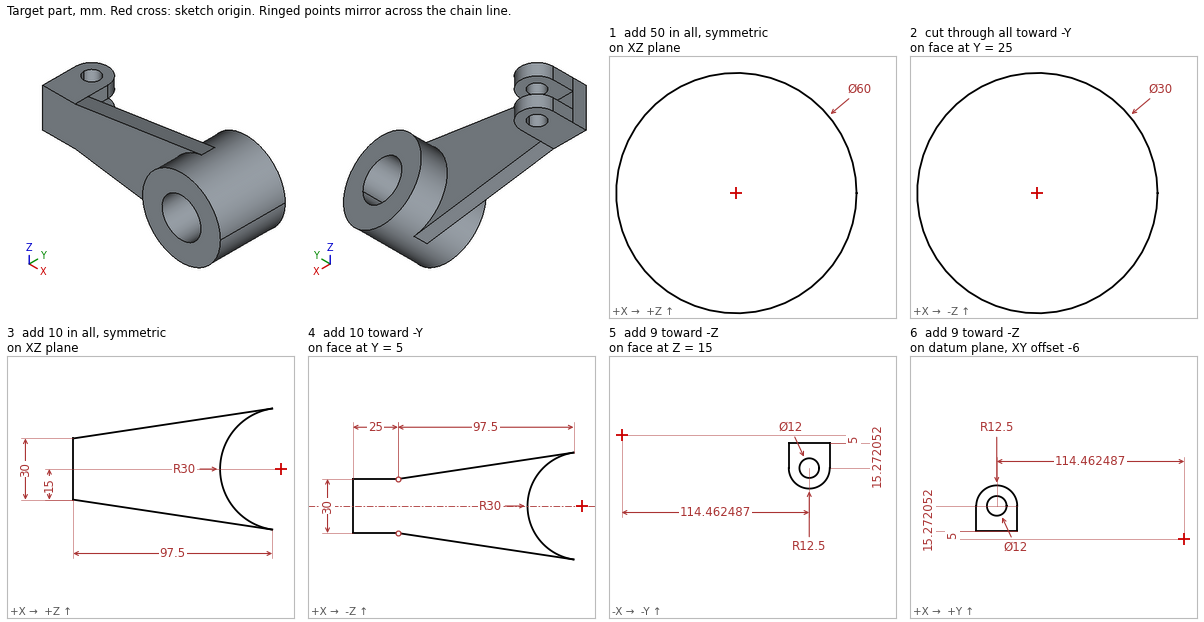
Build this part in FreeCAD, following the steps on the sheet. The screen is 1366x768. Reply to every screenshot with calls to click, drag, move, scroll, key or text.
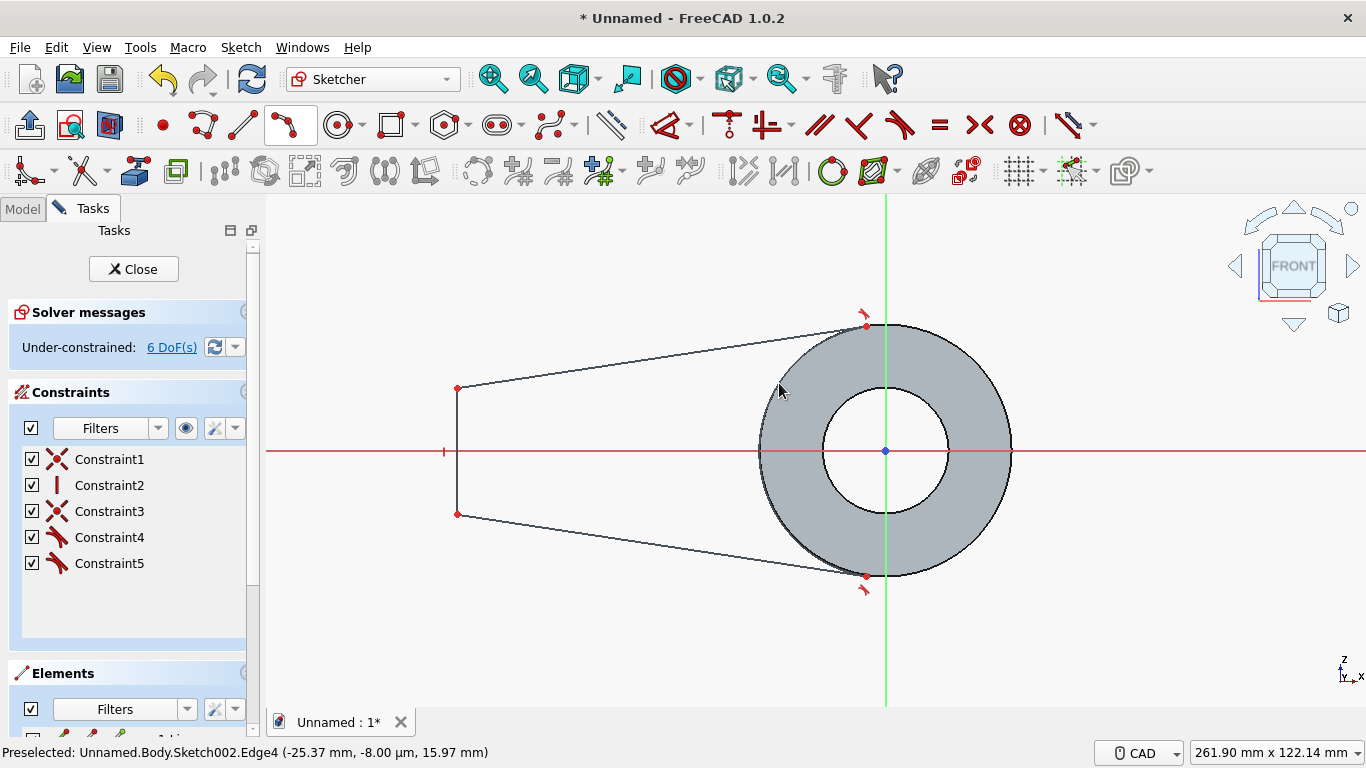
drag(876, 441, 896, 461)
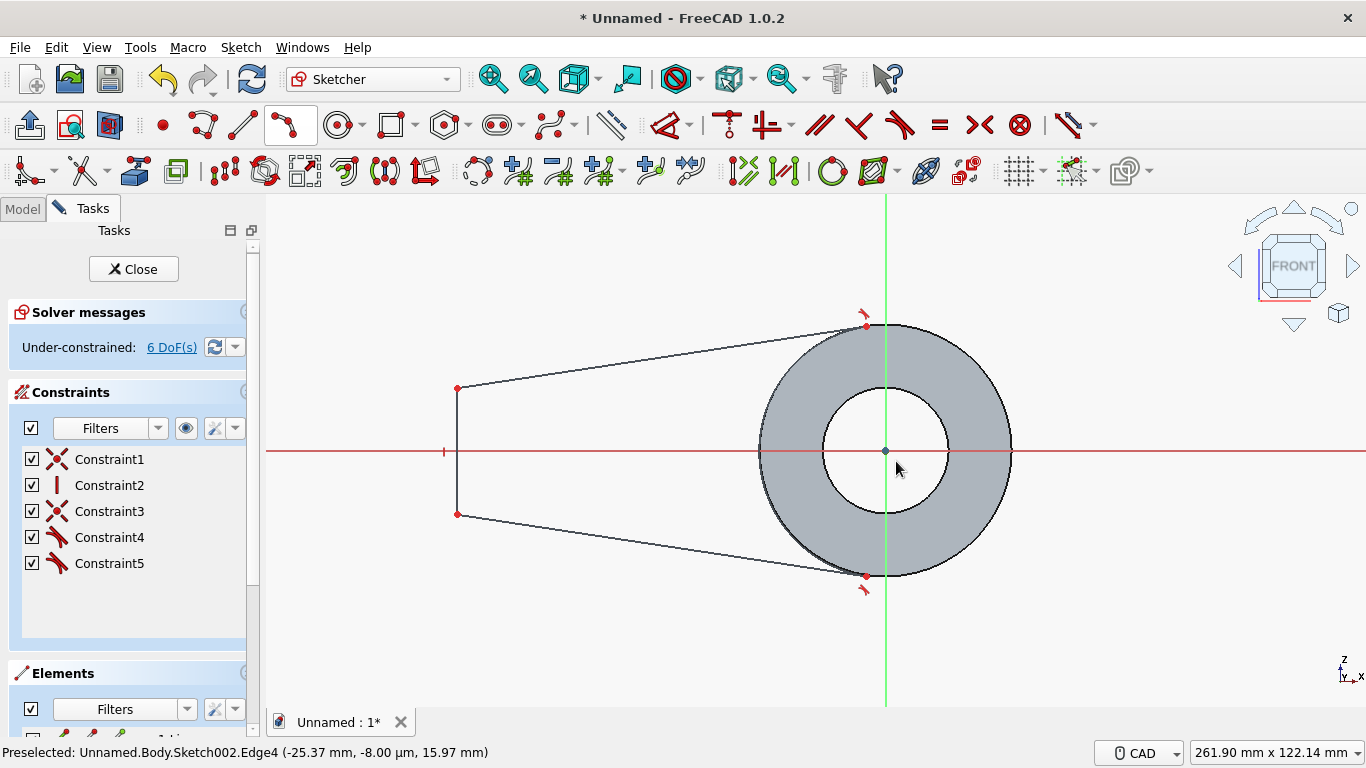
click(728, 126)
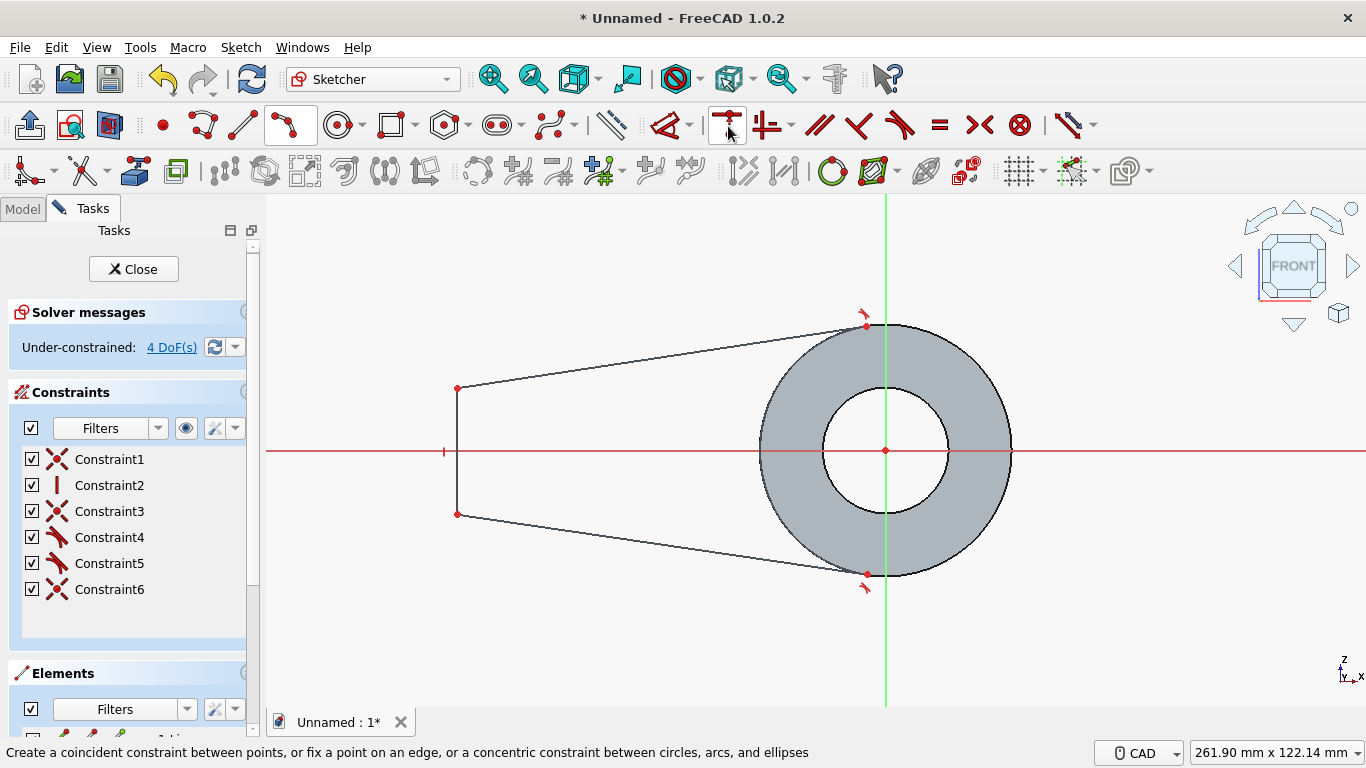
click(780, 383)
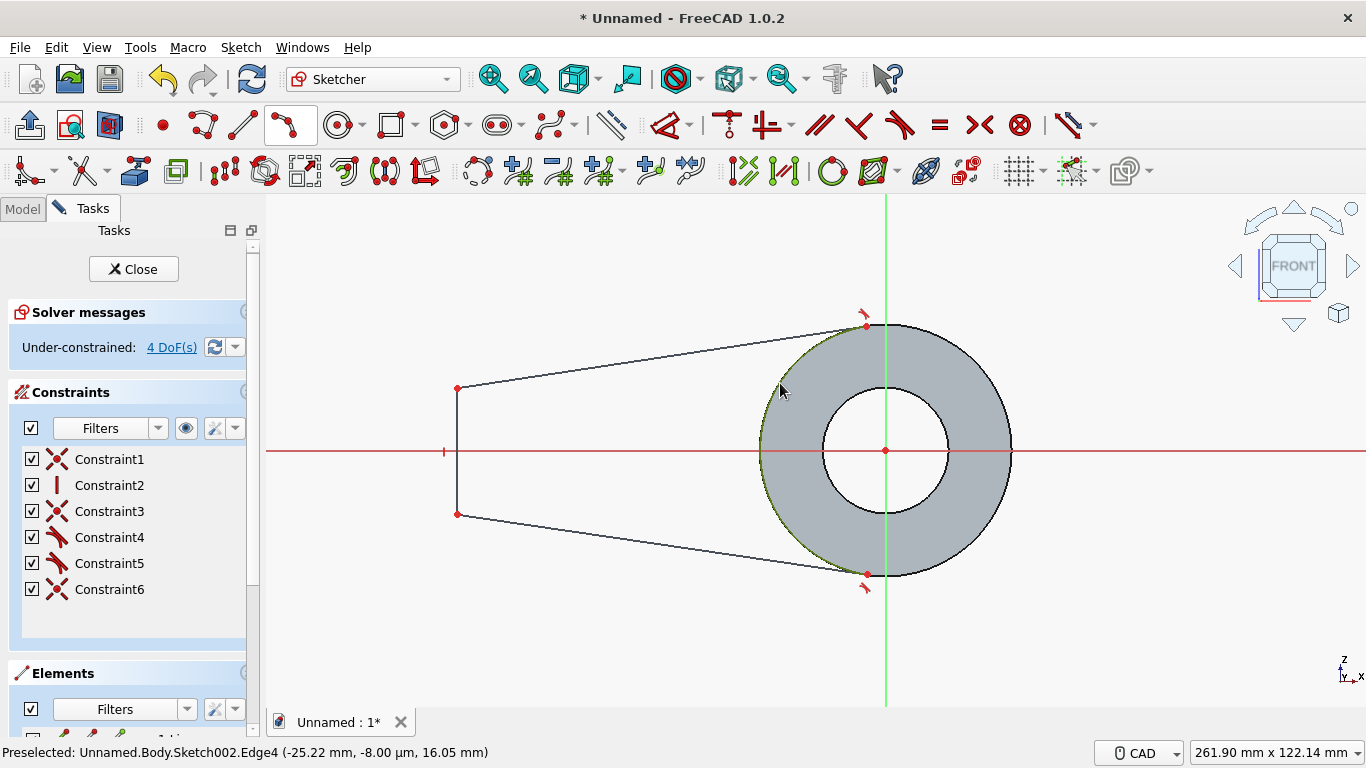
key(k)
key(r)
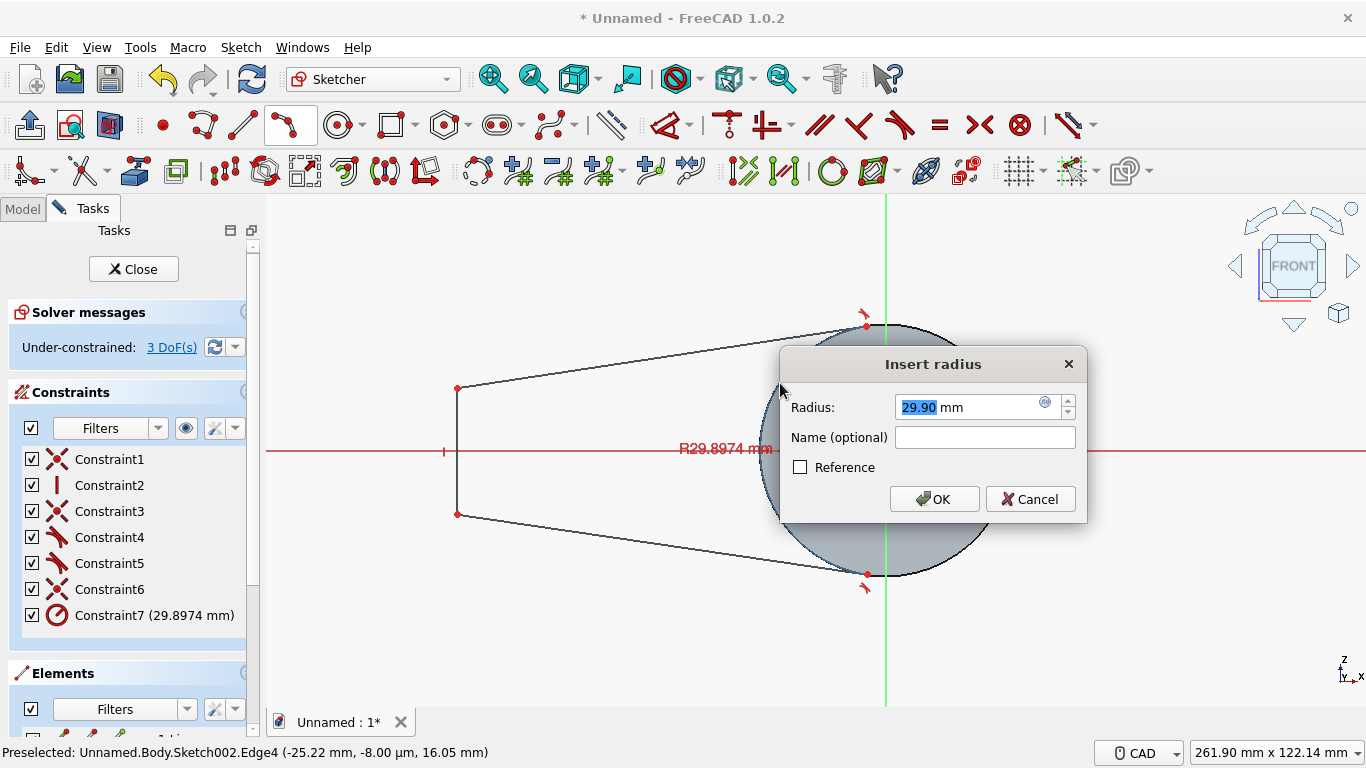
text(30)
key(Return)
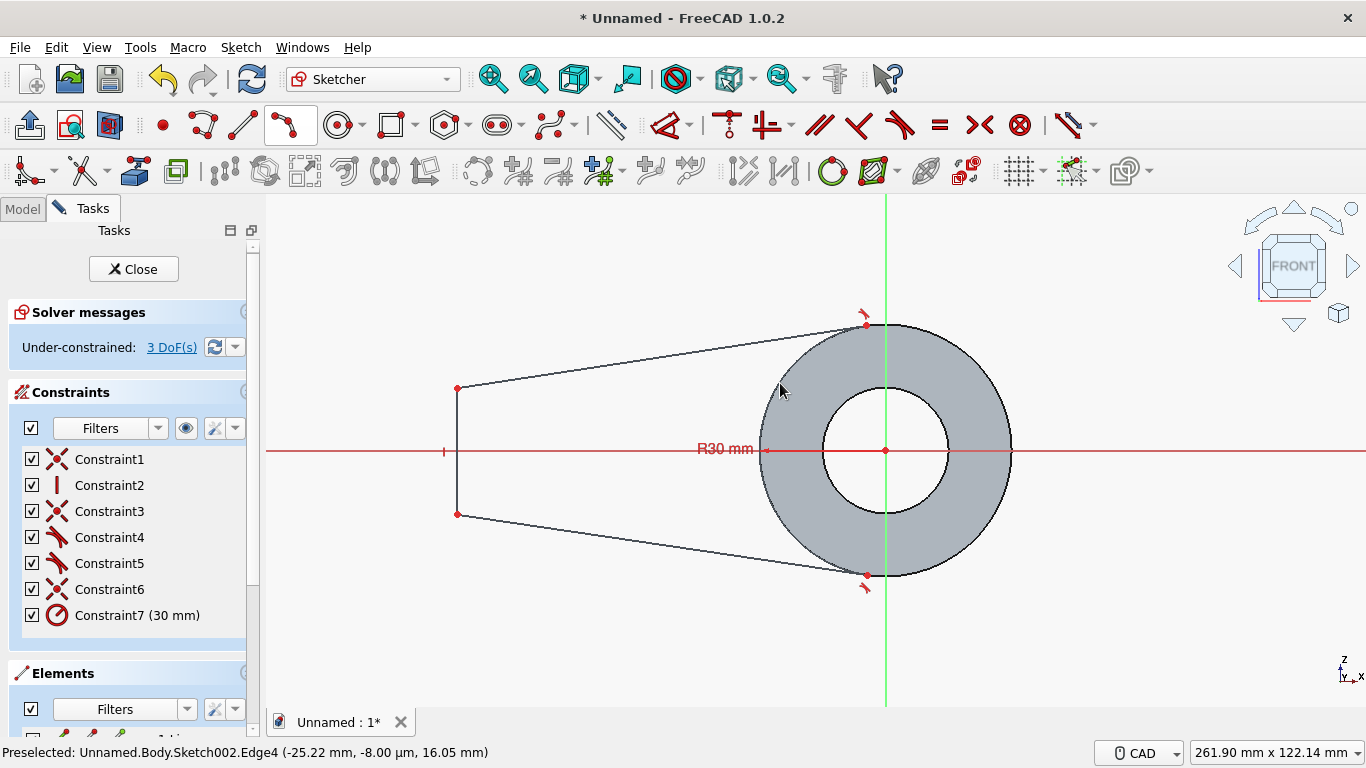
click(457, 477)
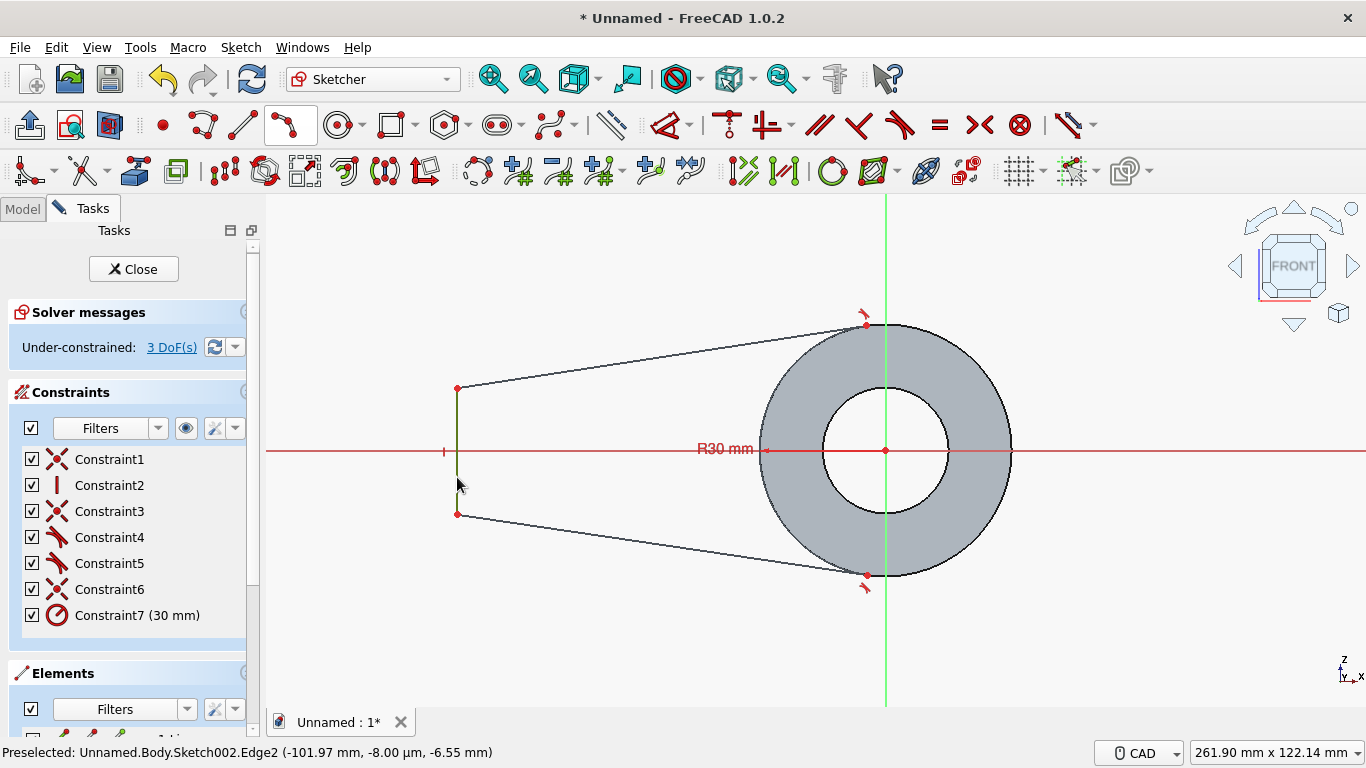
key(i)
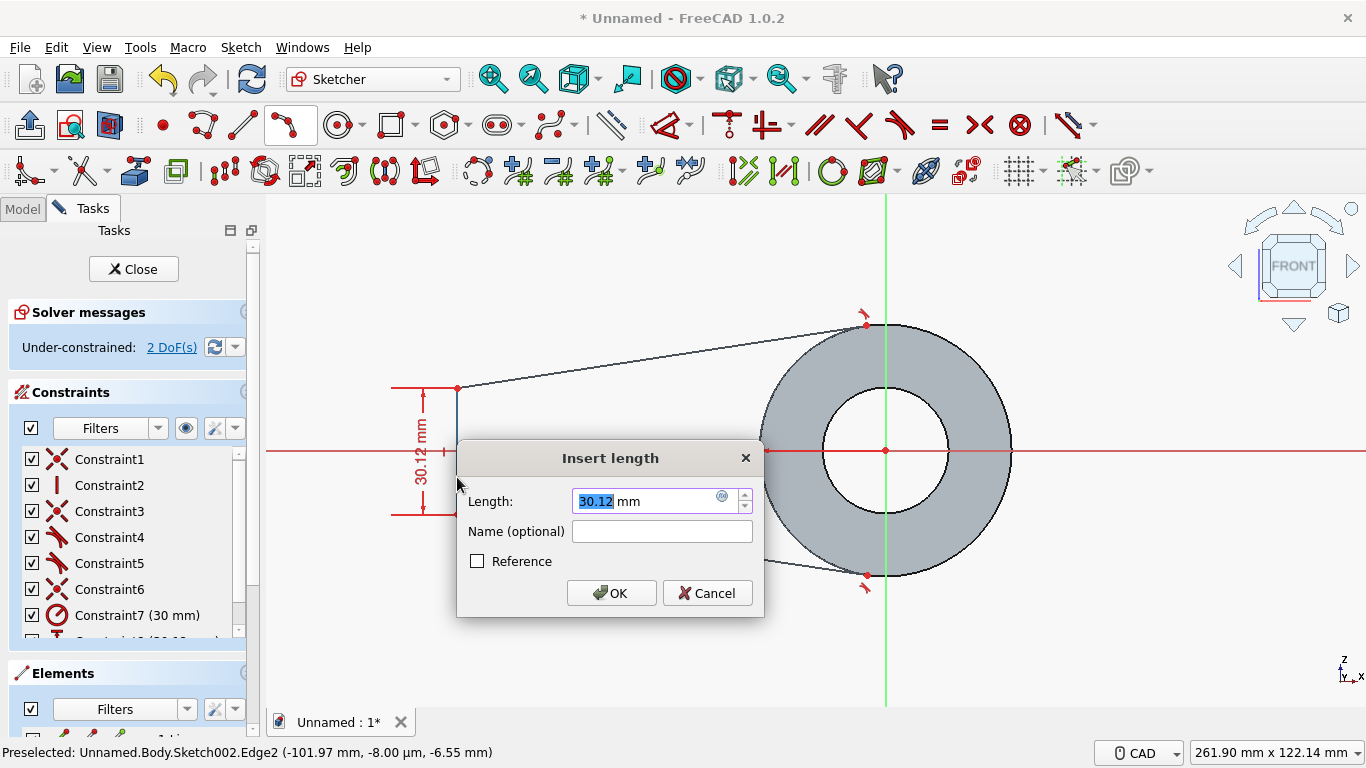
text(30)
key(Return)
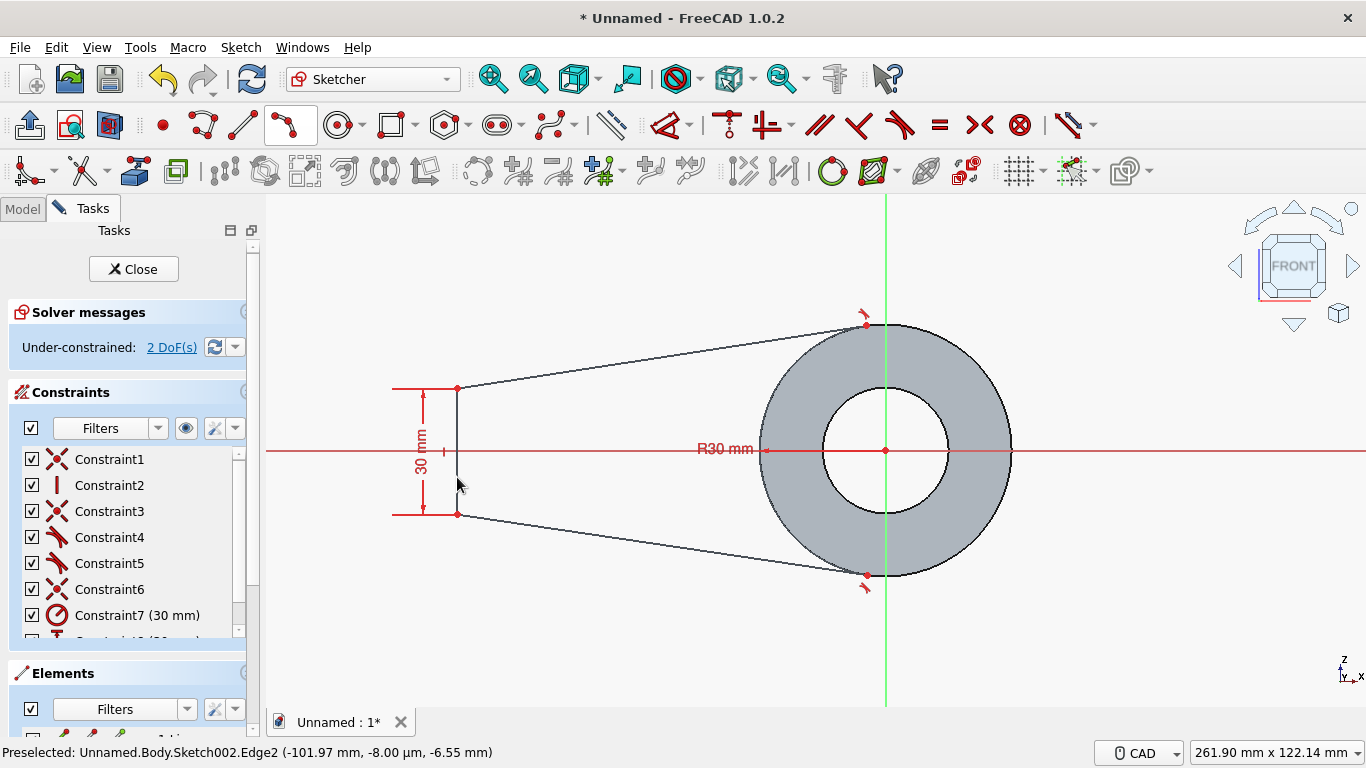
click(457, 515)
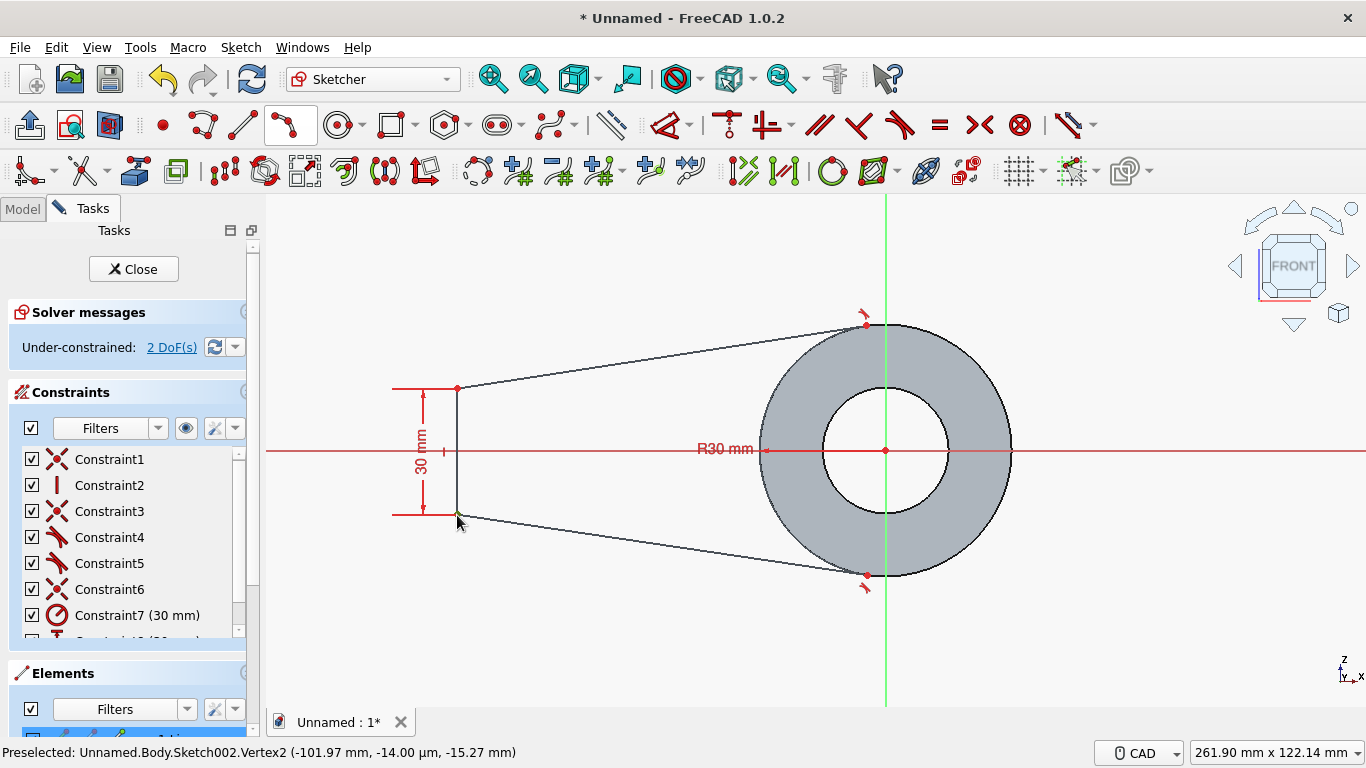
key(i)